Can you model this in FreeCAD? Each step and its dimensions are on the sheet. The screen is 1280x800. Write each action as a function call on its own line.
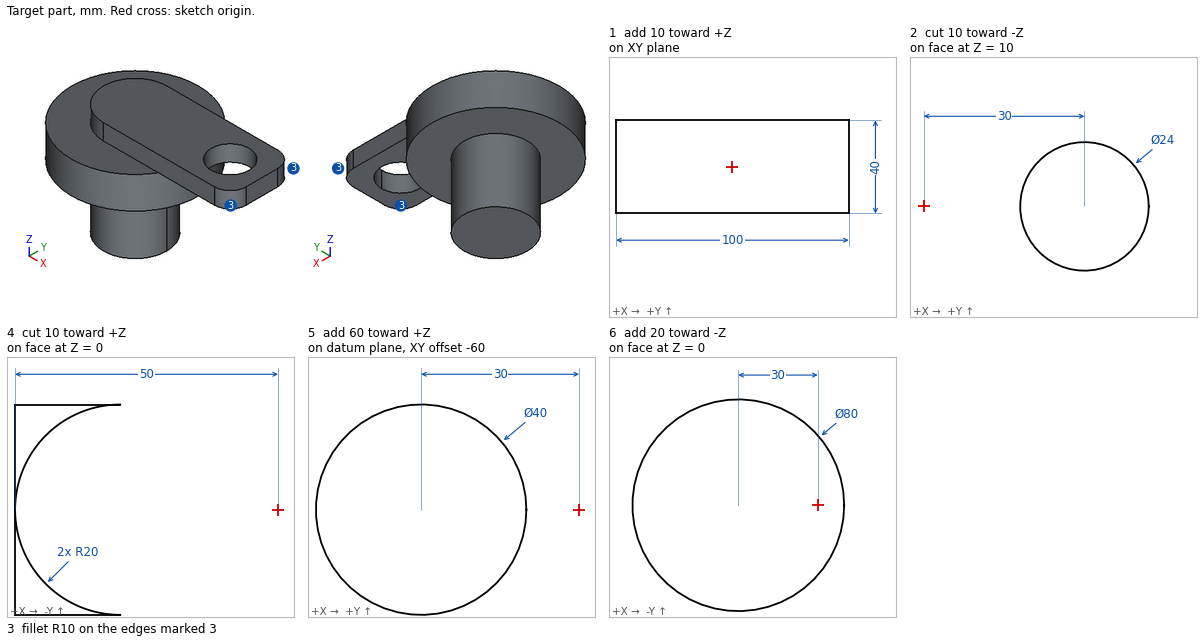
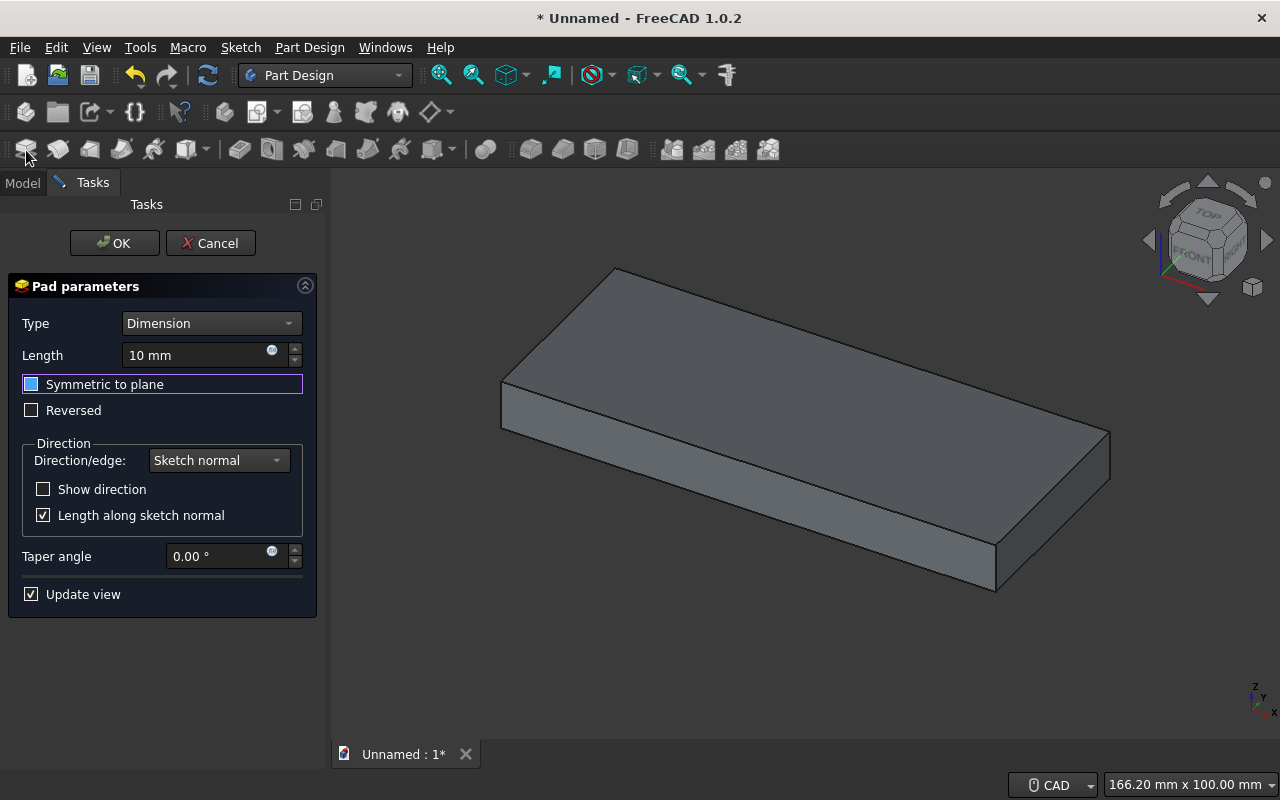
click(115, 243)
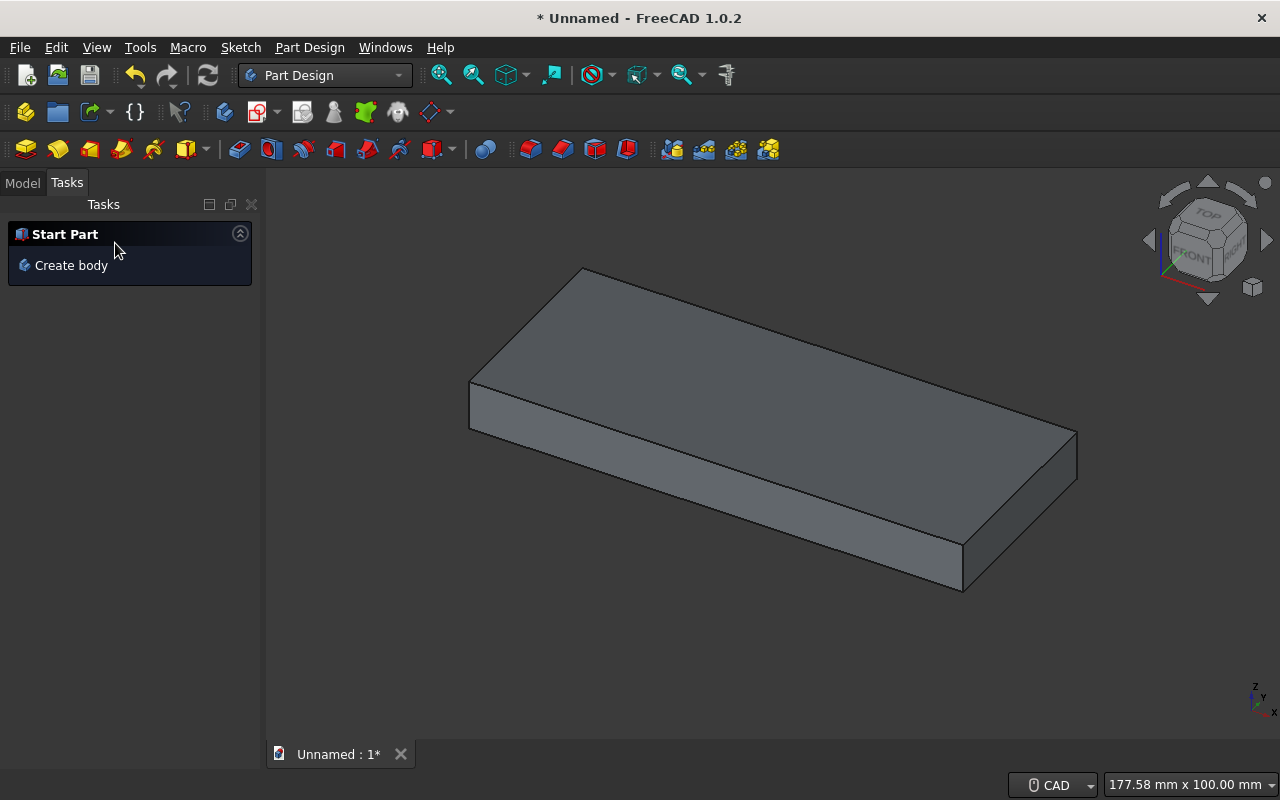
click(914, 453)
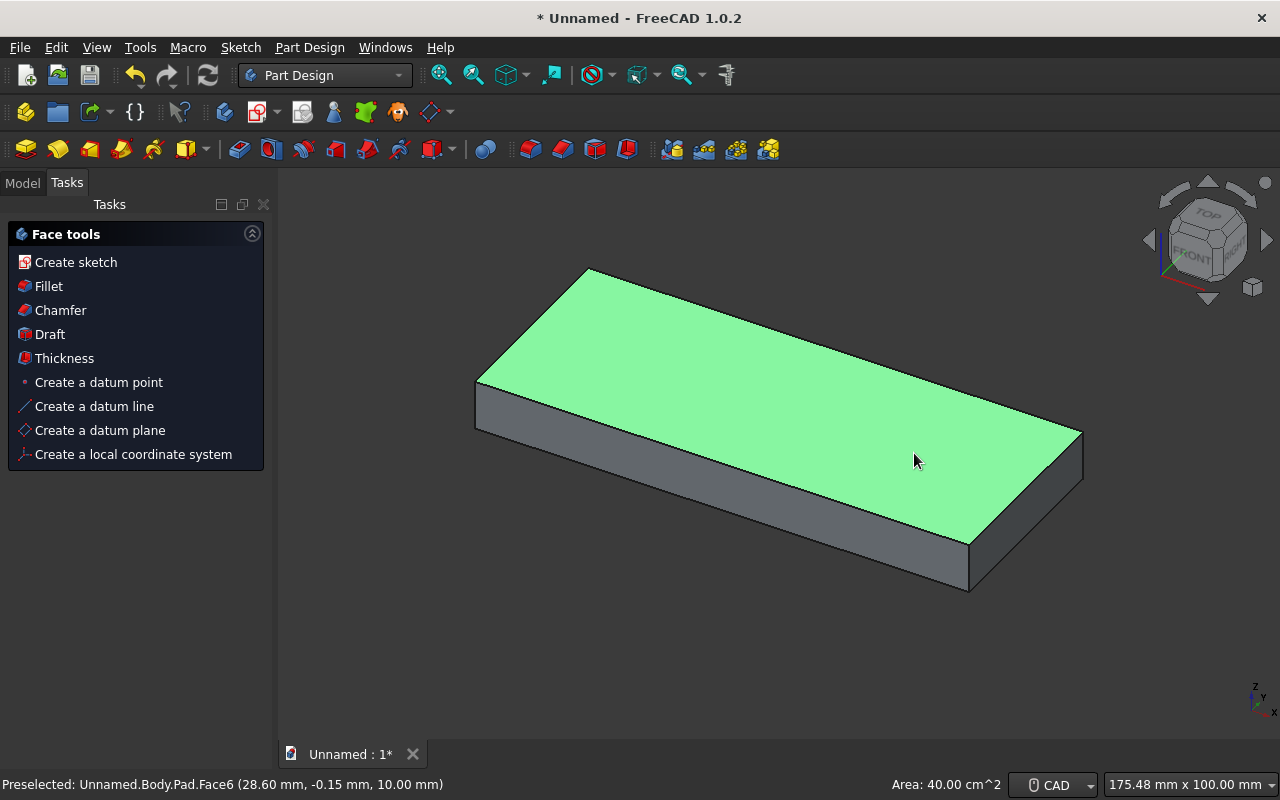
click(258, 112)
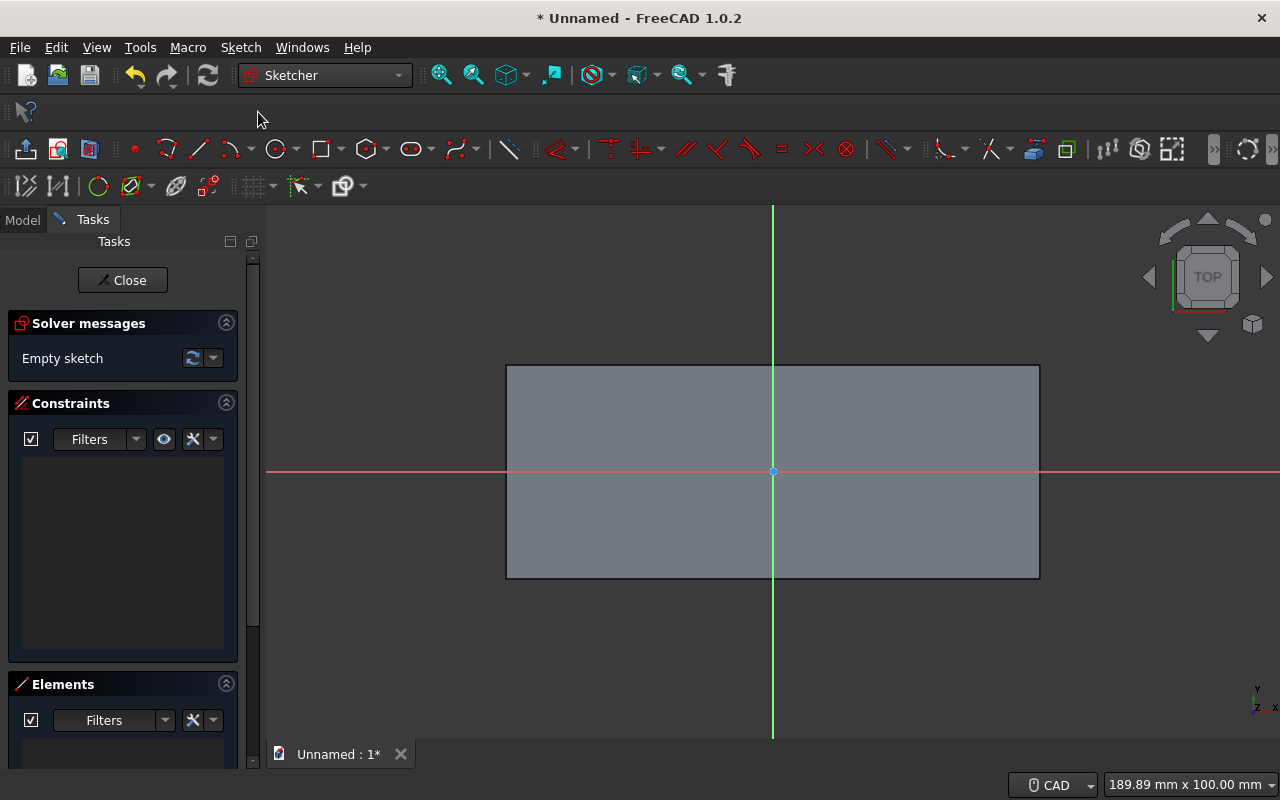
scroll(990, 472, up, 5)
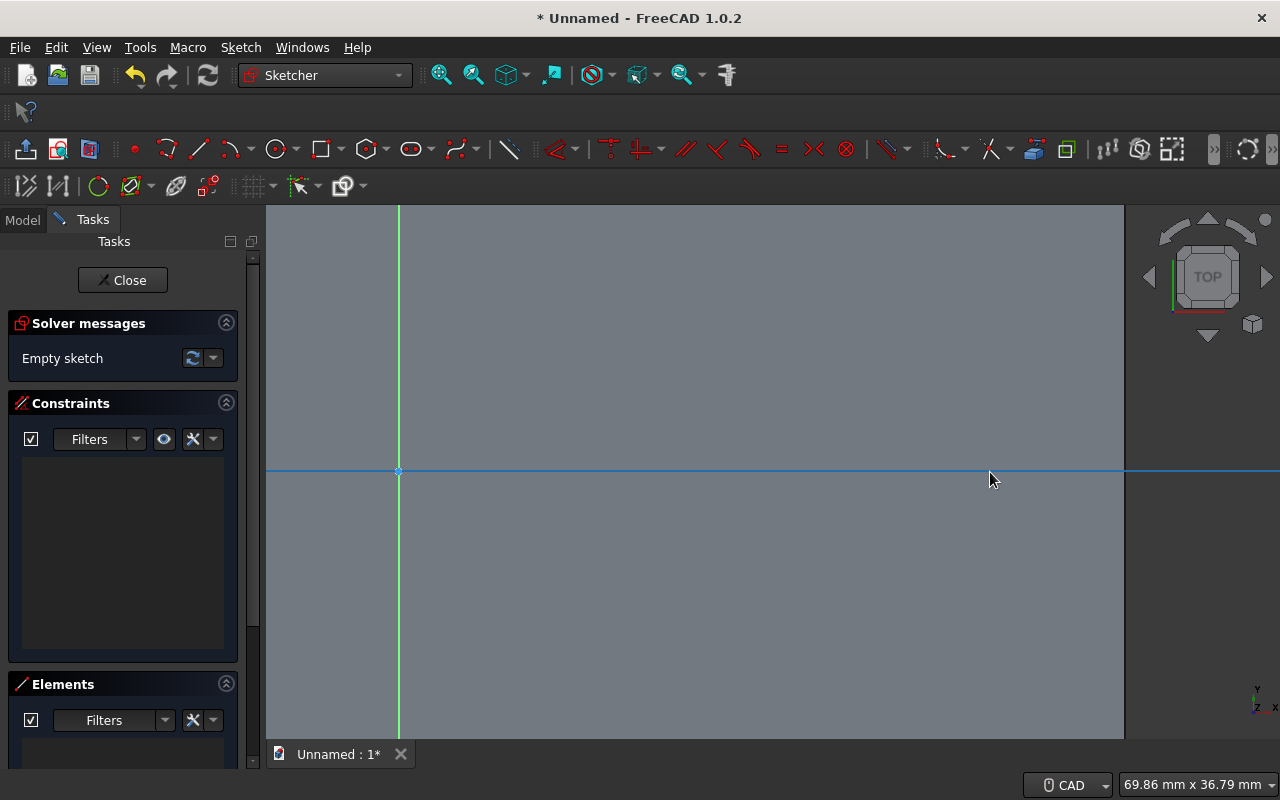
click(276, 150)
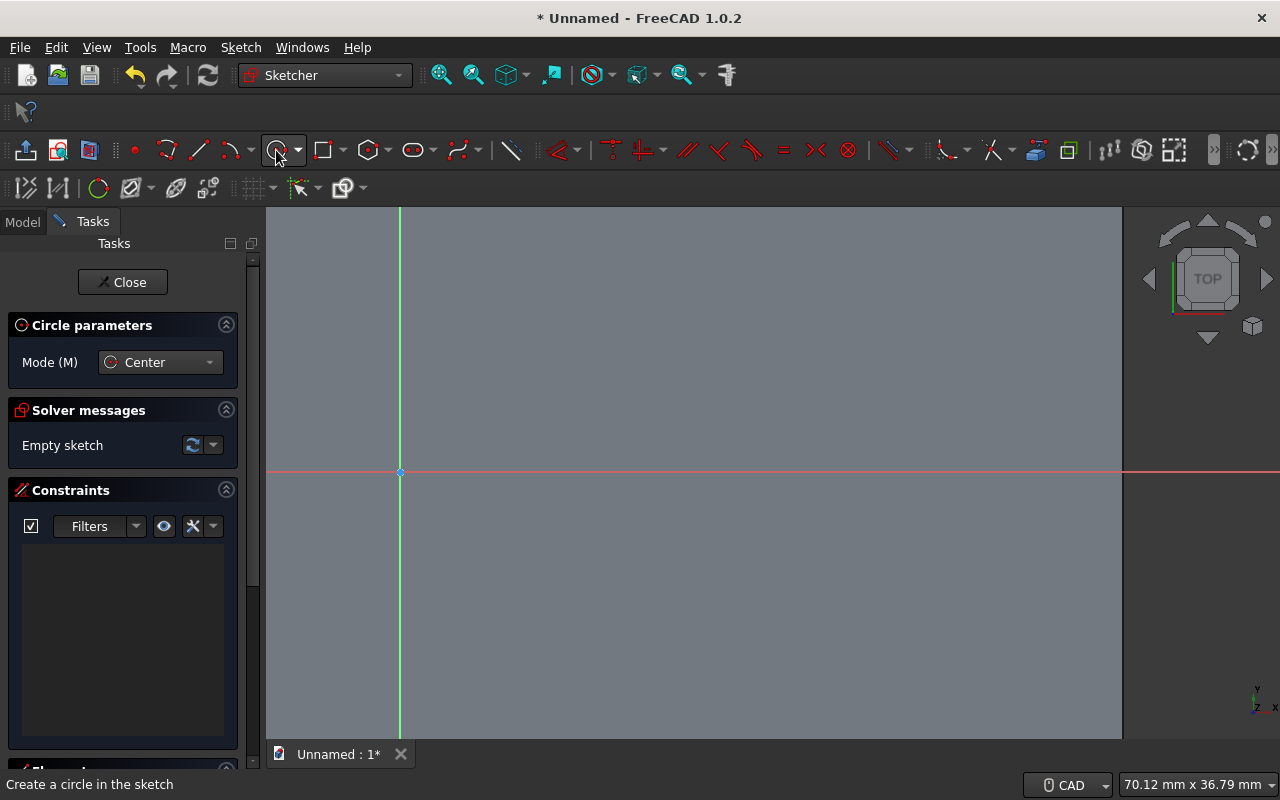
click(834, 472)
move(957, 349)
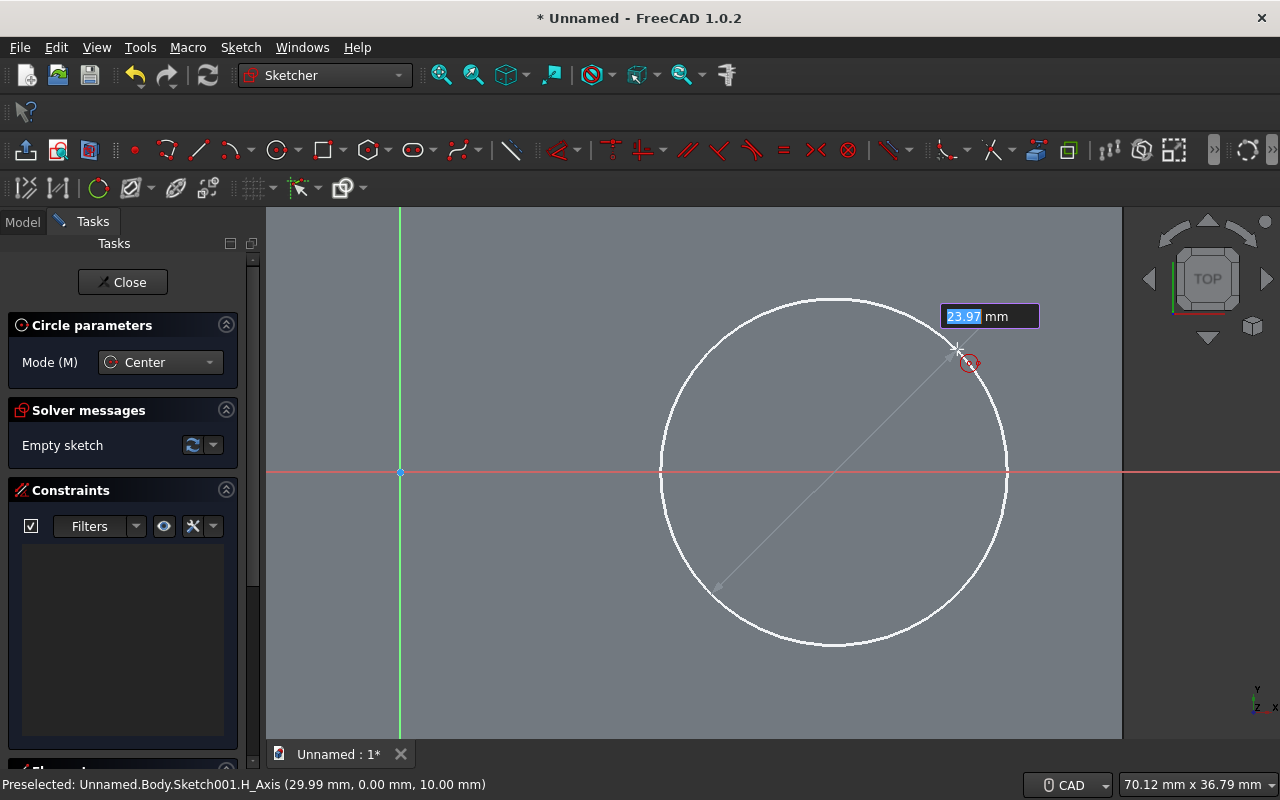
text(24)
key(Return)
key(Escape)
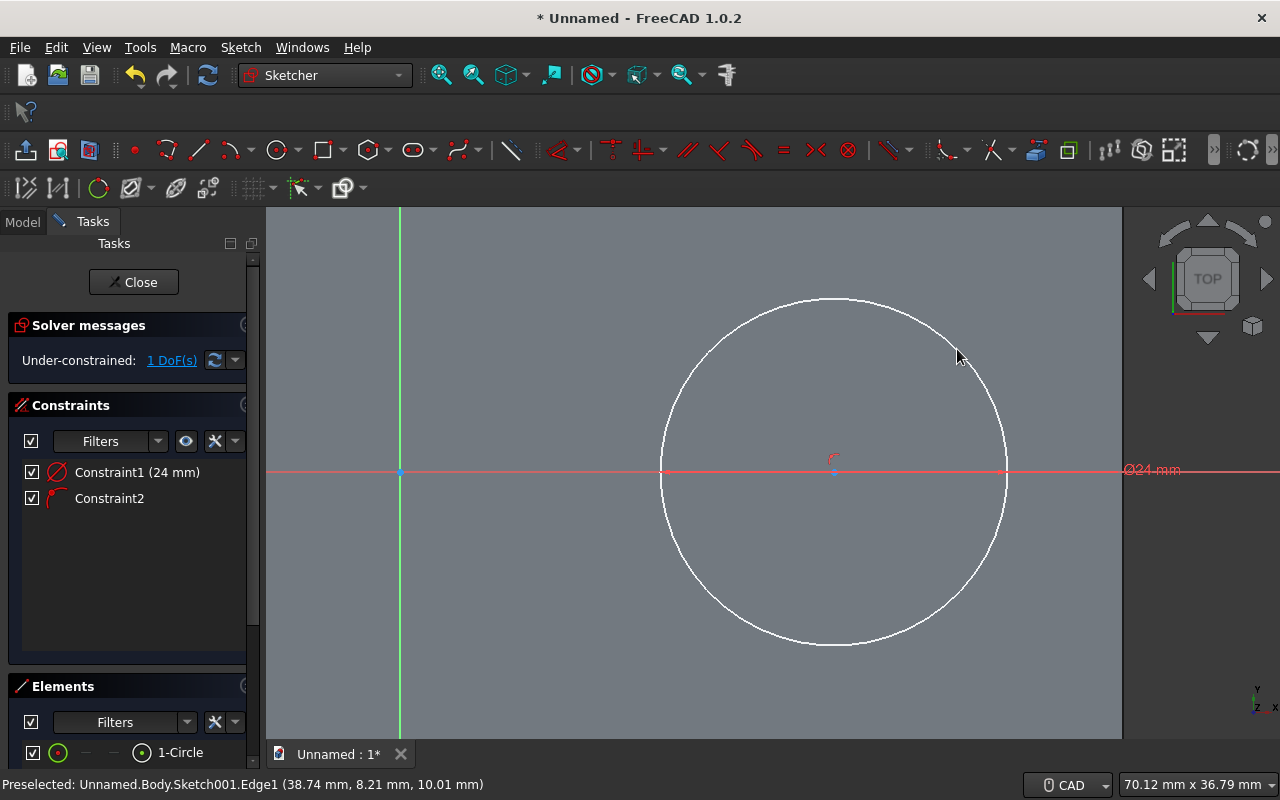
click(834, 472)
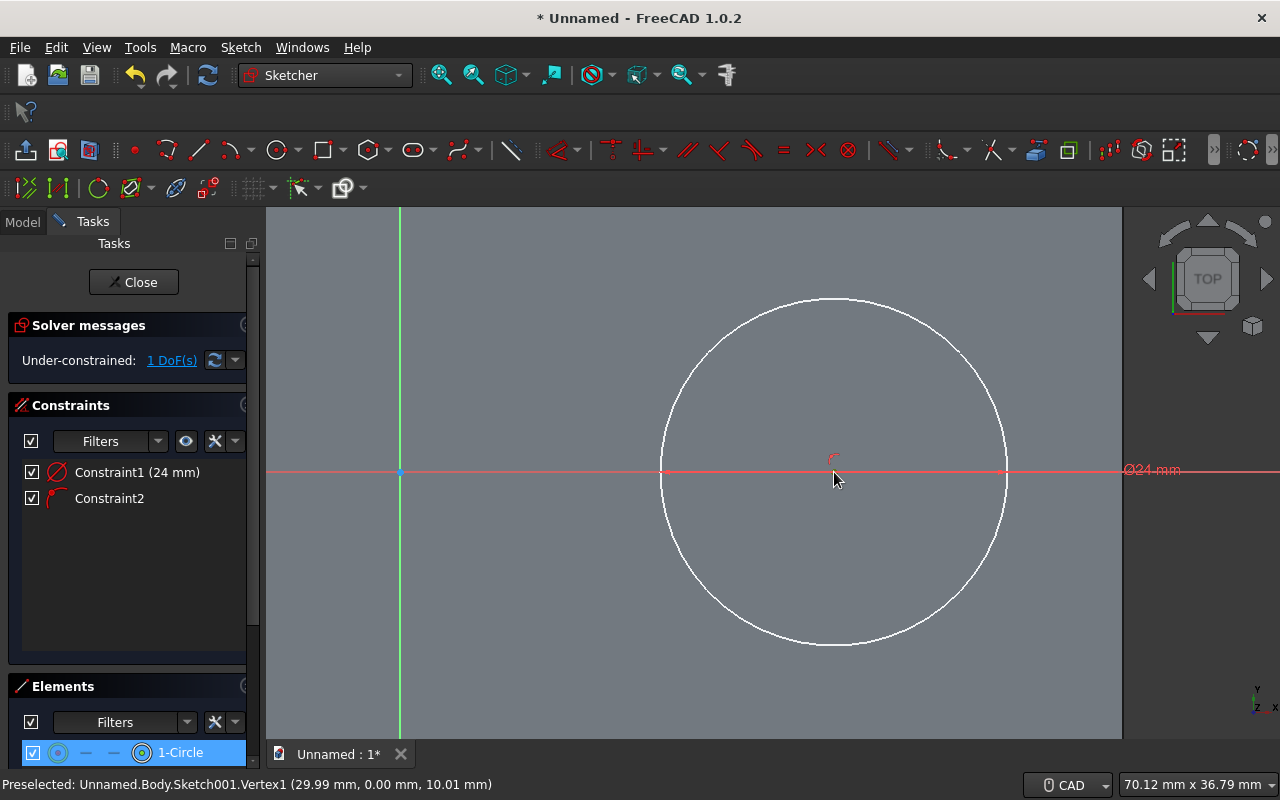
key(l)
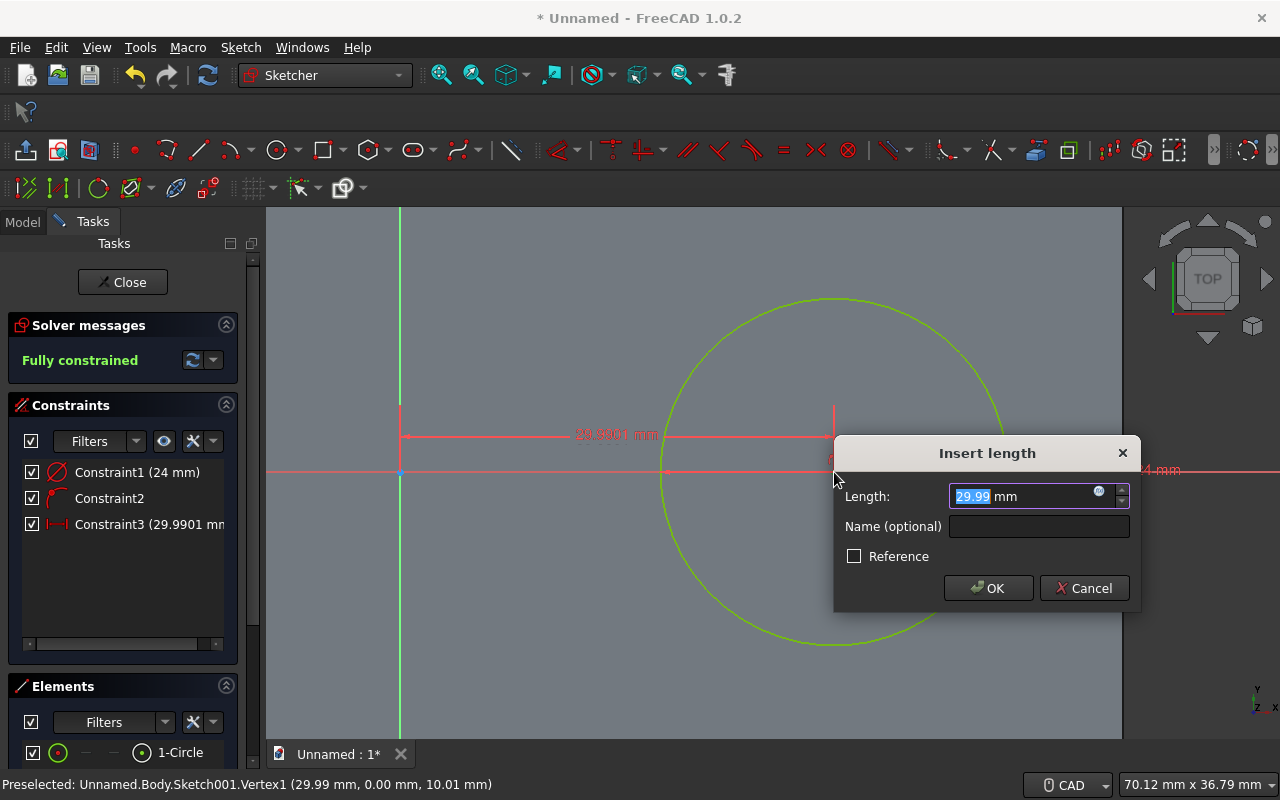
text(30)
key(Return)